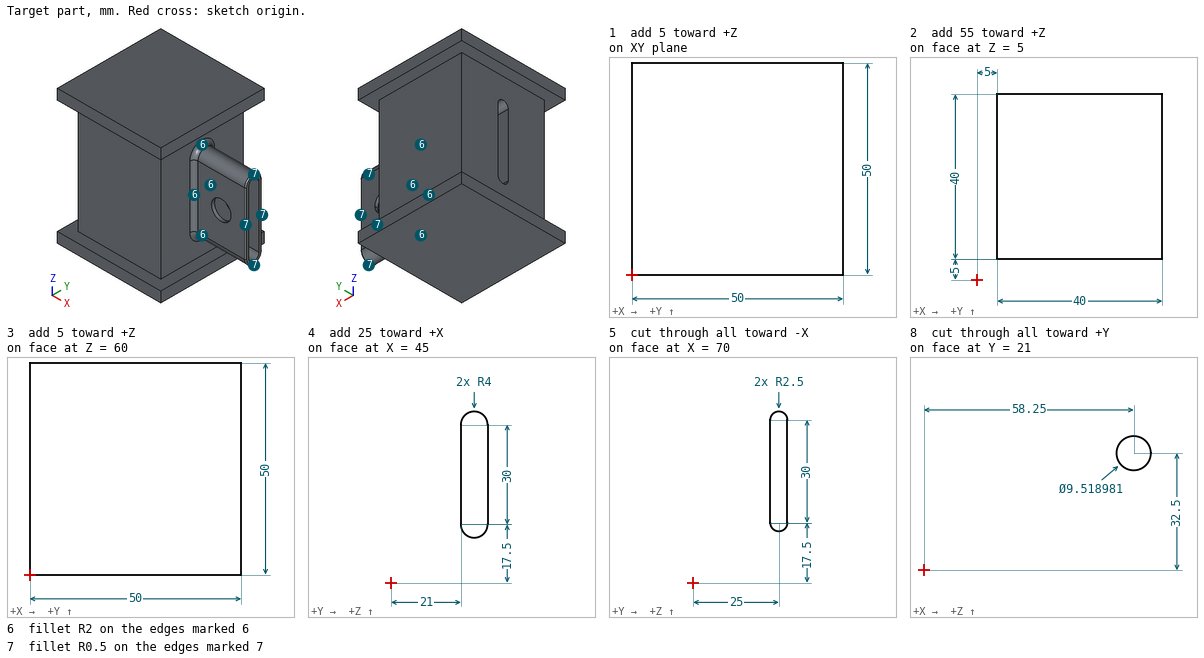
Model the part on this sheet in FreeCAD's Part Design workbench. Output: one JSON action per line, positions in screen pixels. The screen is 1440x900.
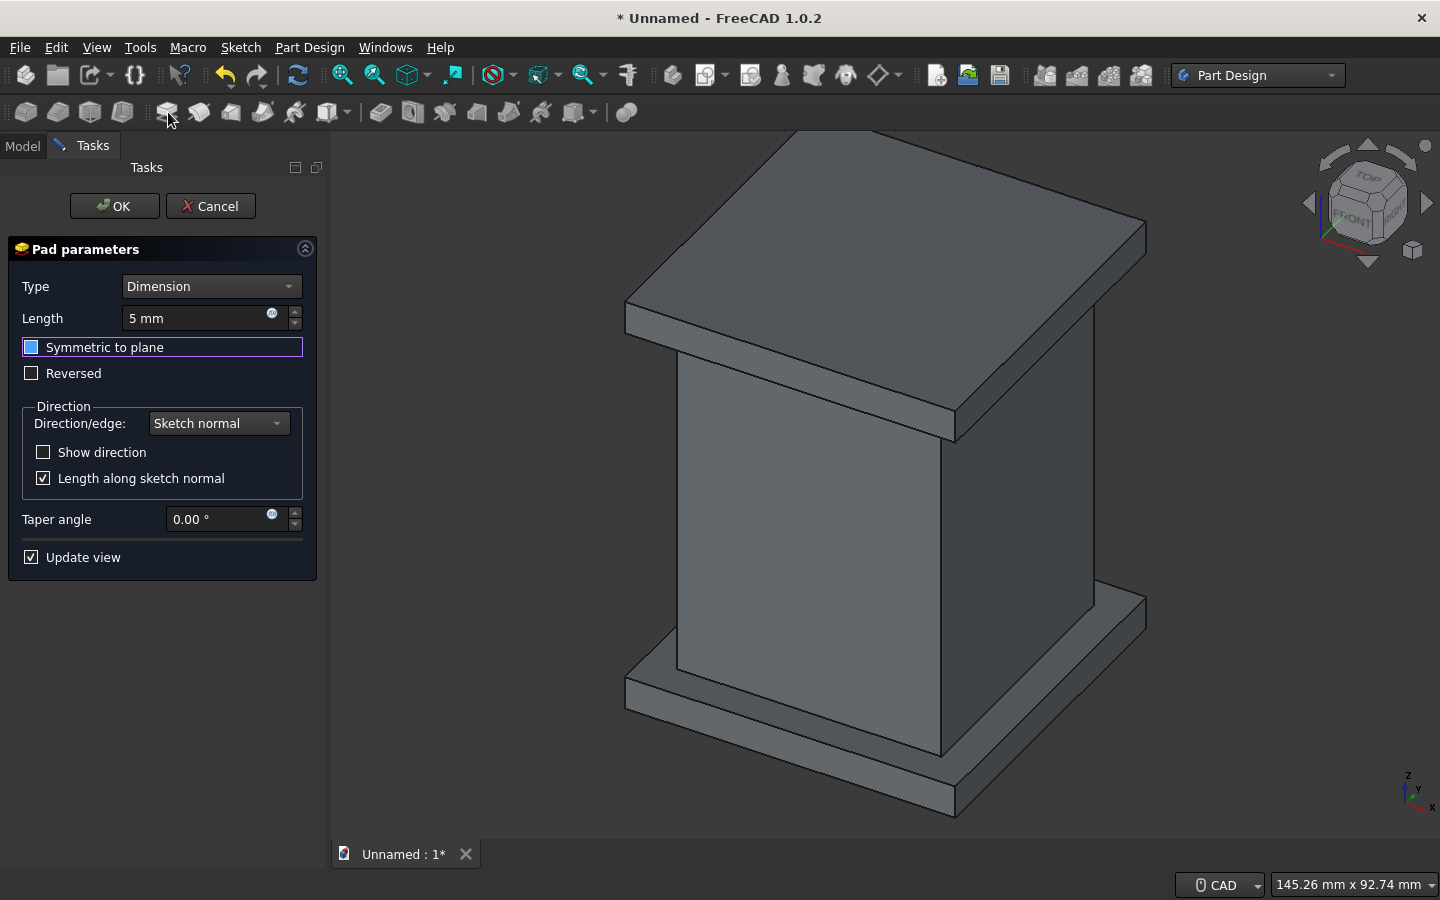
{"action": "left_click", "coordinate": [115, 206]}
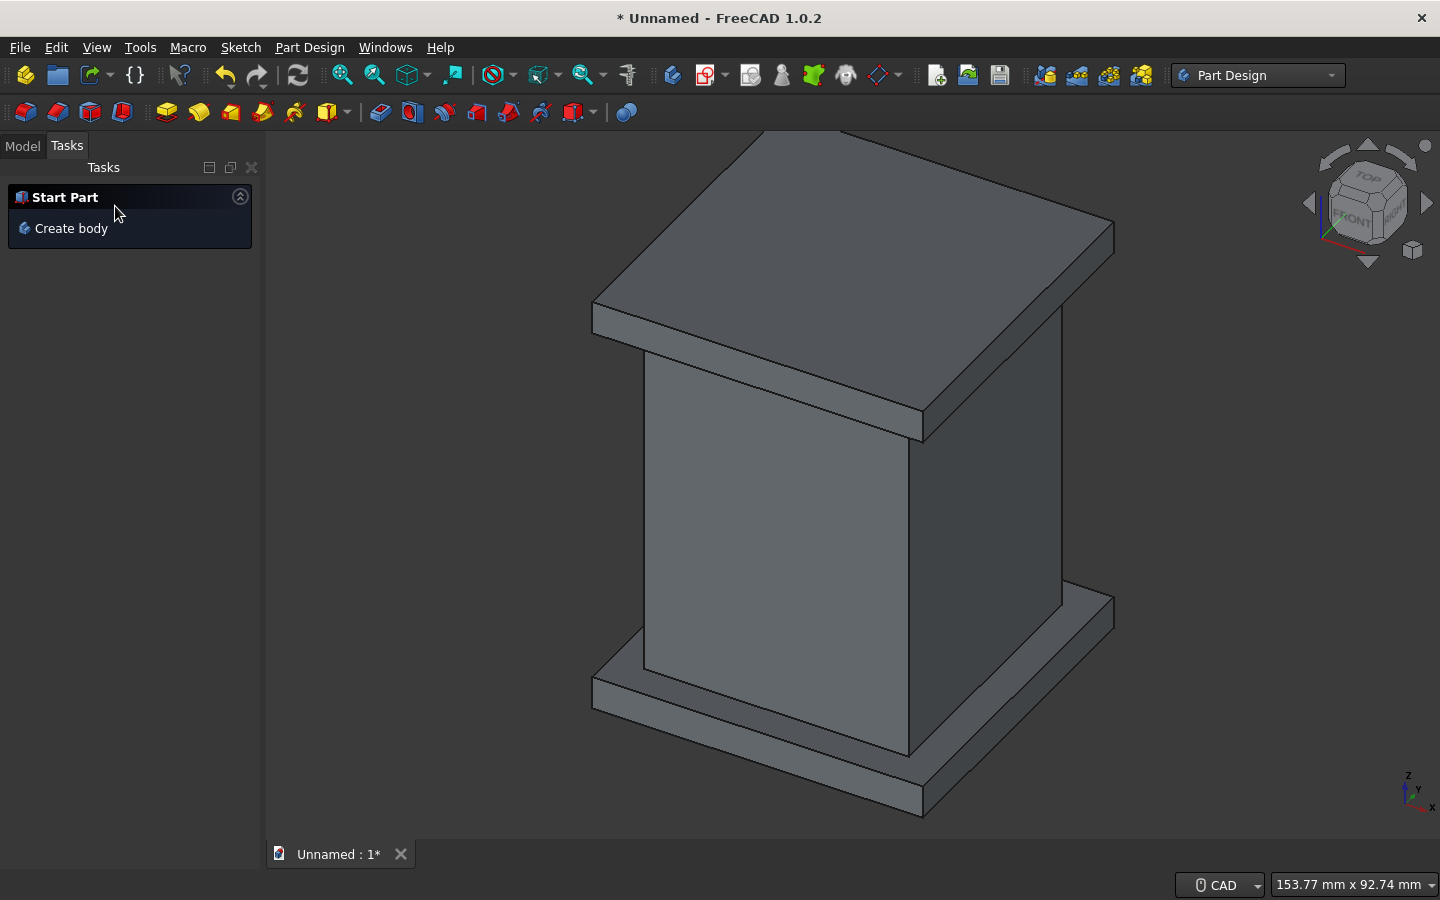
{"action": "left_click", "coordinate": [344, 76]}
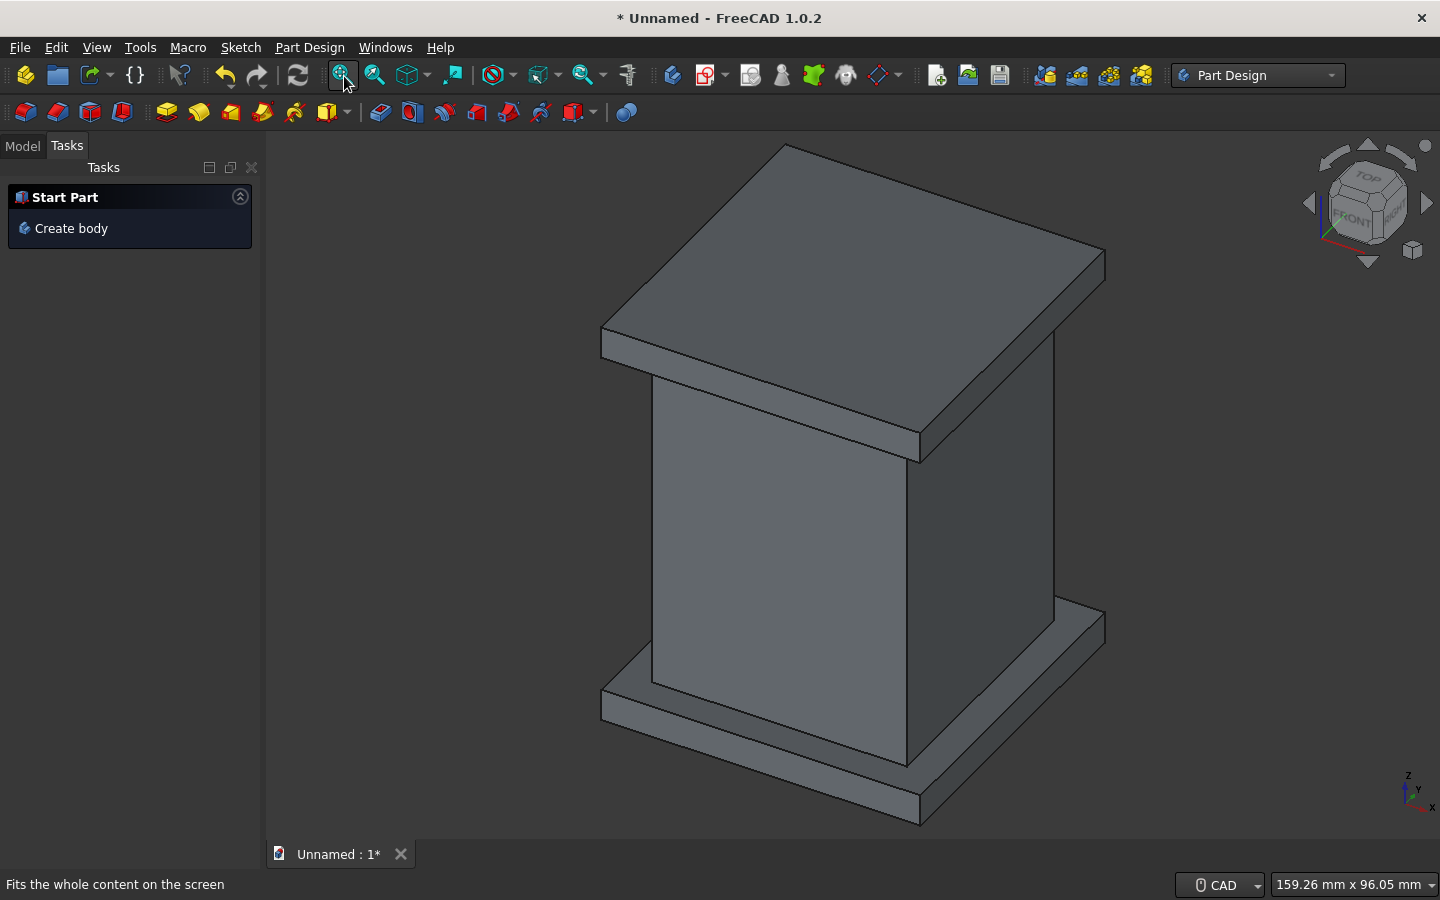
{"action": "left_click", "coordinate": [981, 526]}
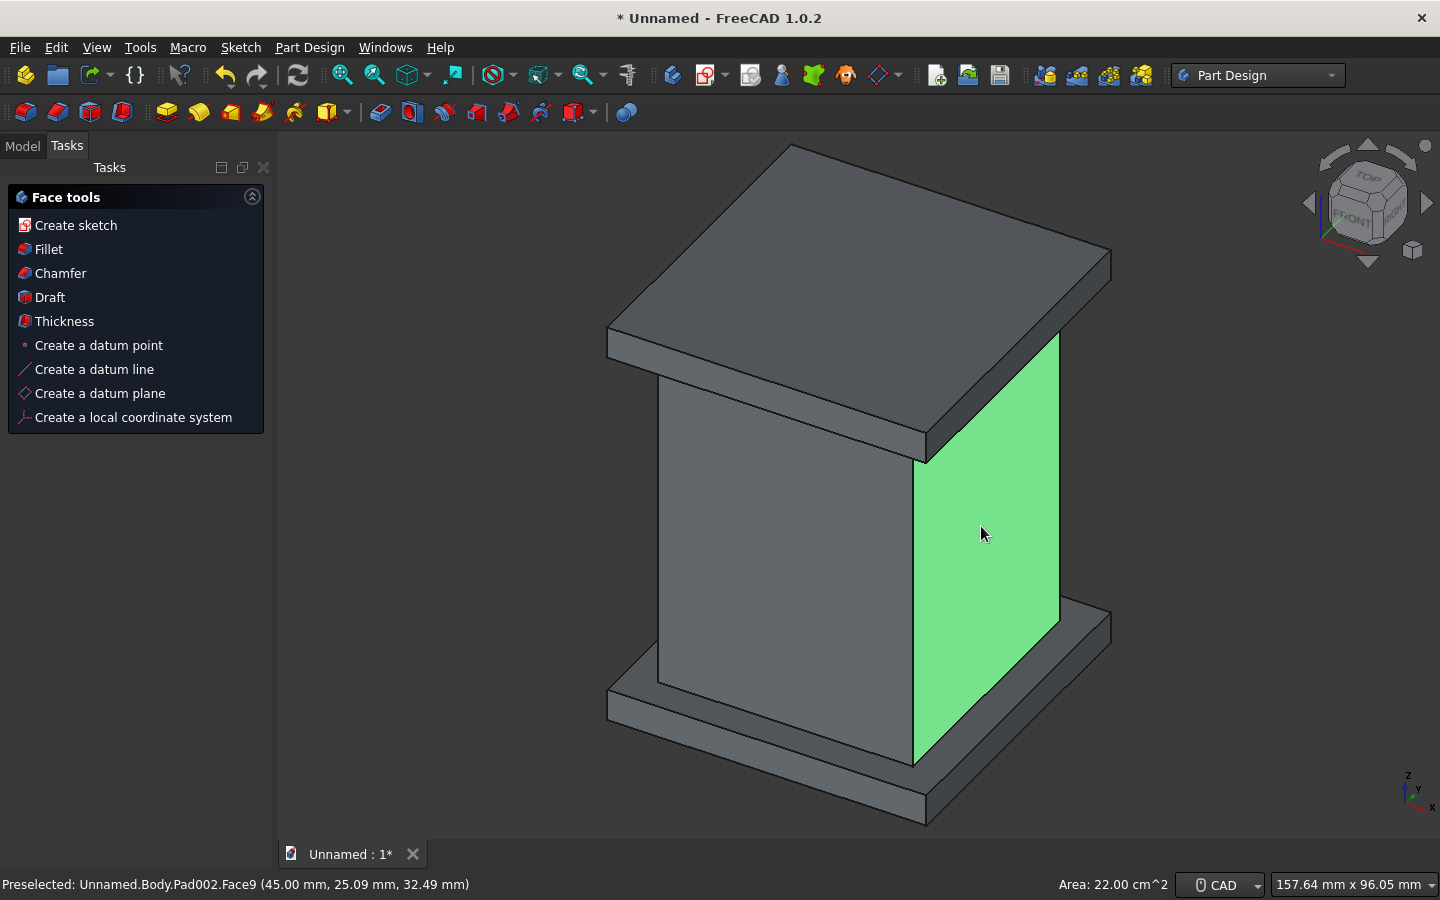
{"action": "left_click", "coordinate": [706, 76]}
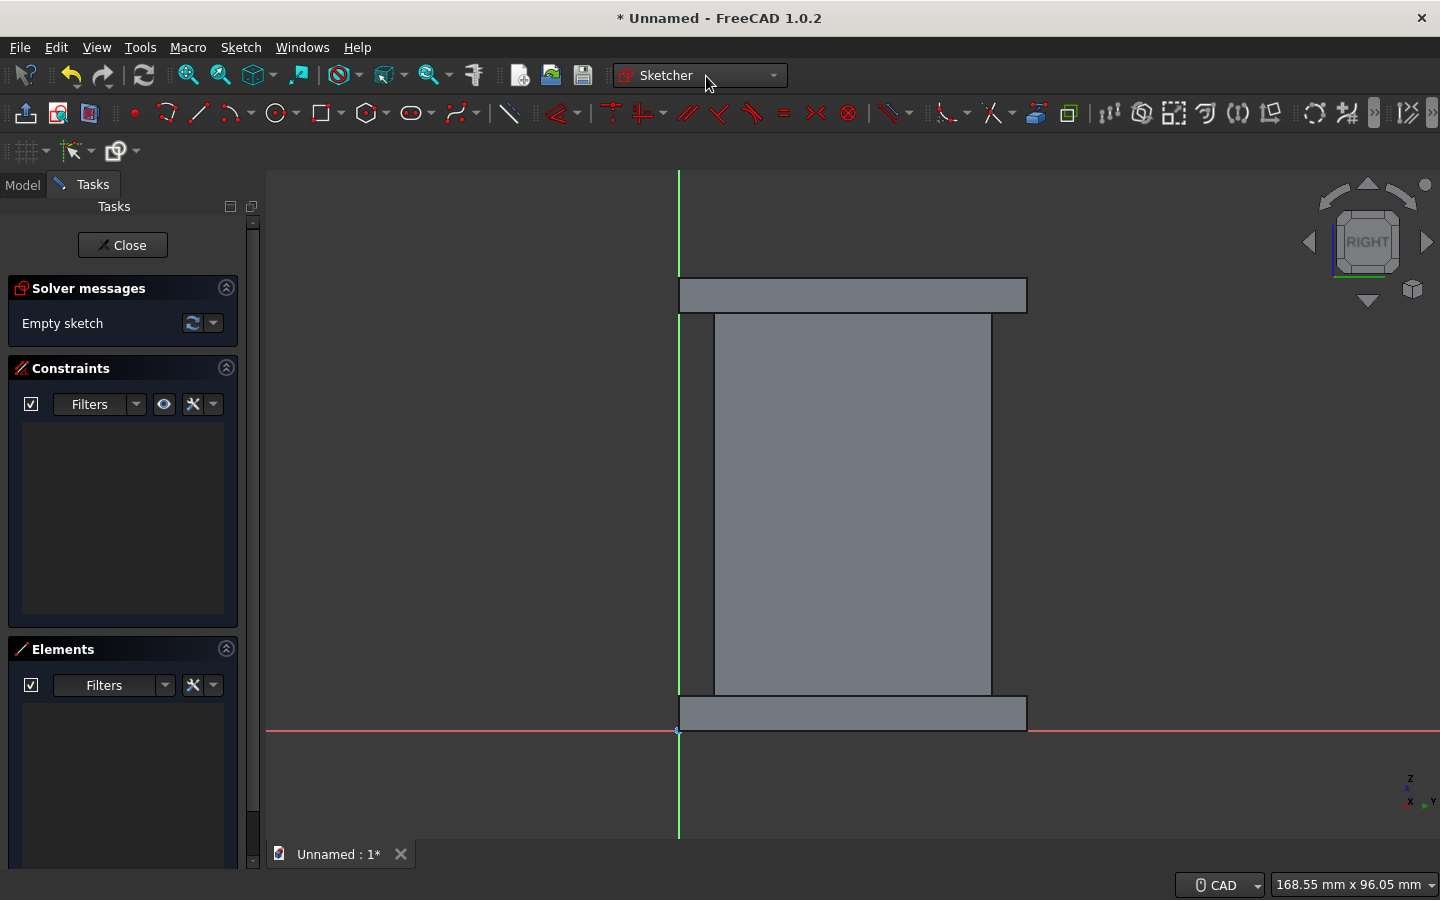
{"action": "left_click", "coordinate": [412, 114]}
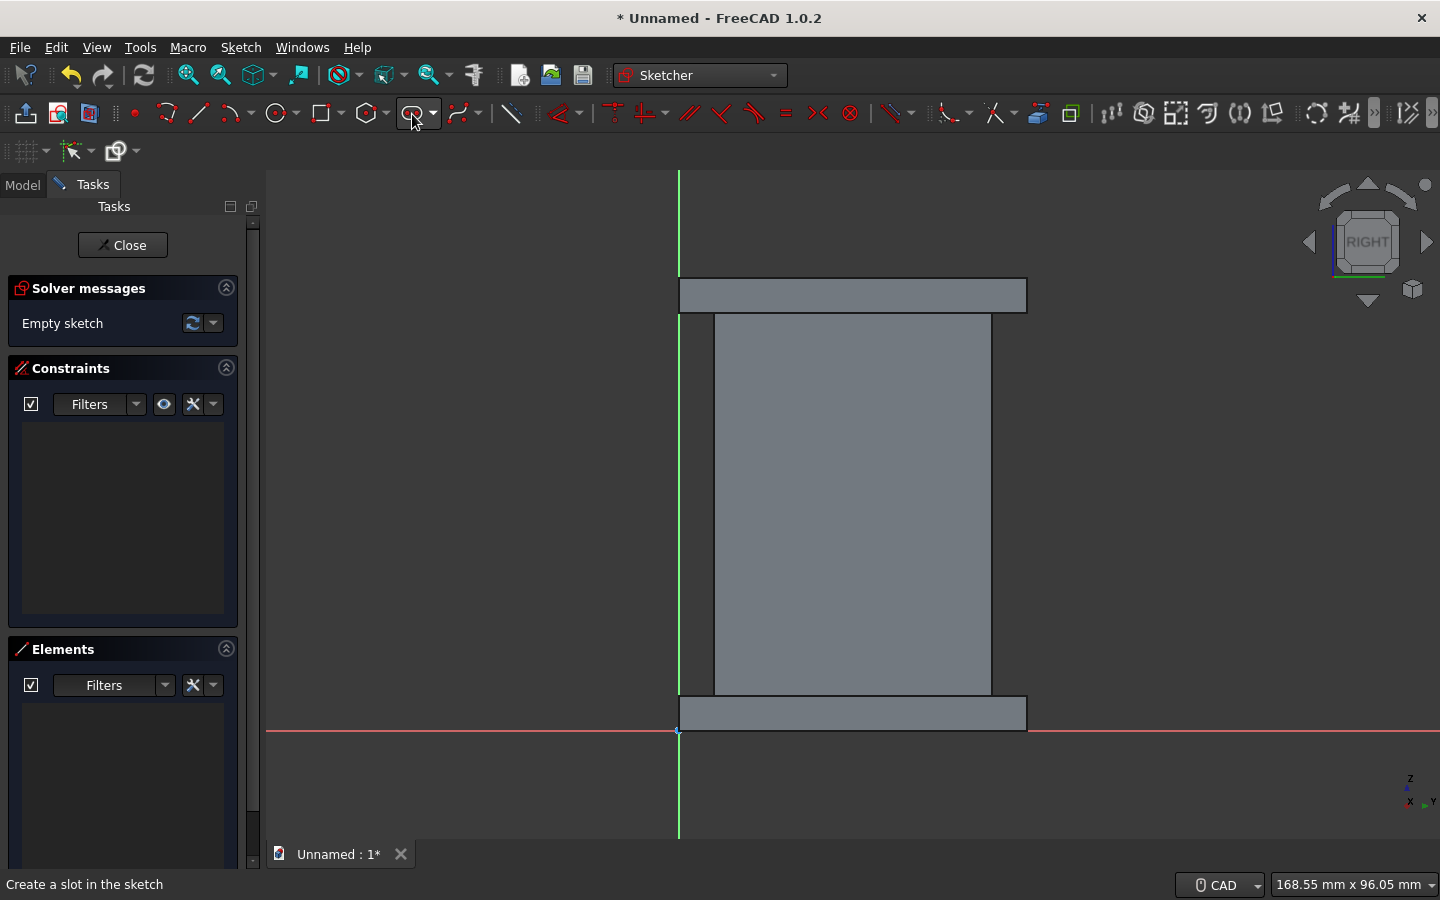
{"action": "left_click", "coordinate": [853, 609]}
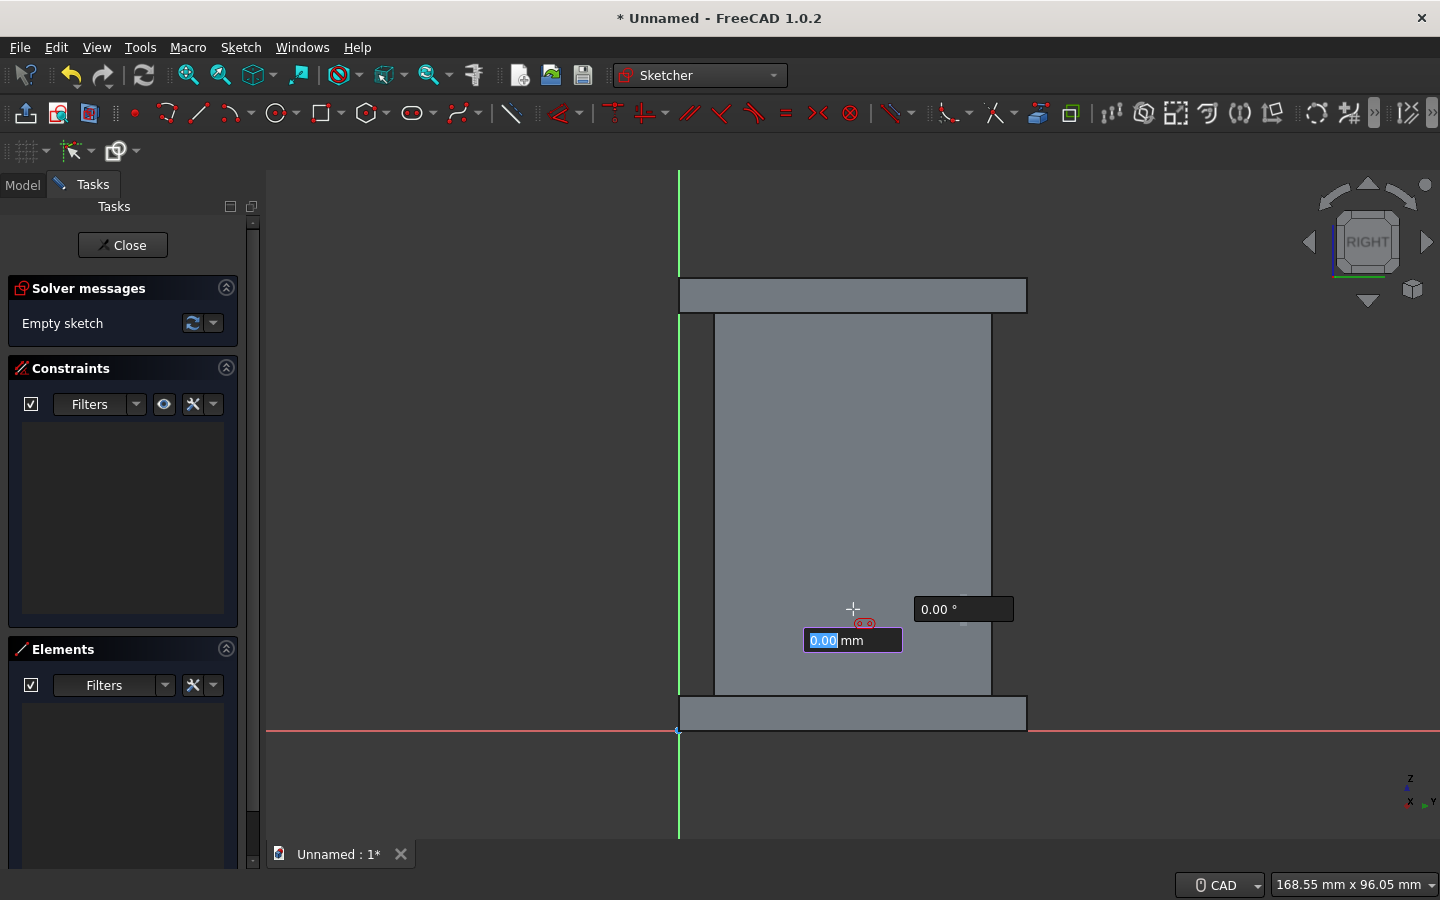
{"action": "left_click", "coordinate": [853, 400]}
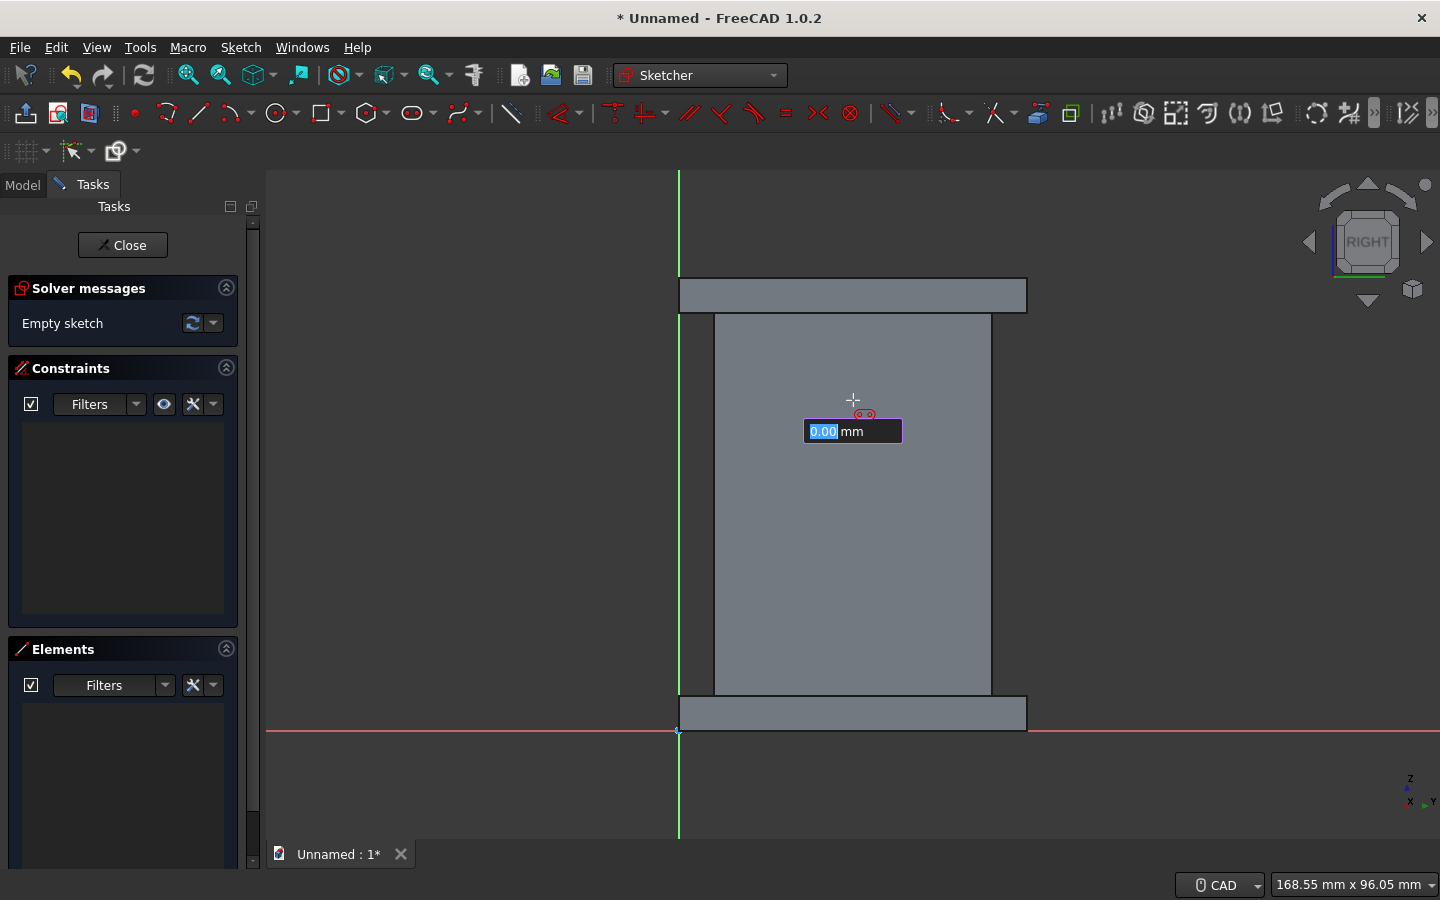
{"action": "left_click", "coordinate": [881, 504]}
{"action": "key", "text": "Escape"}